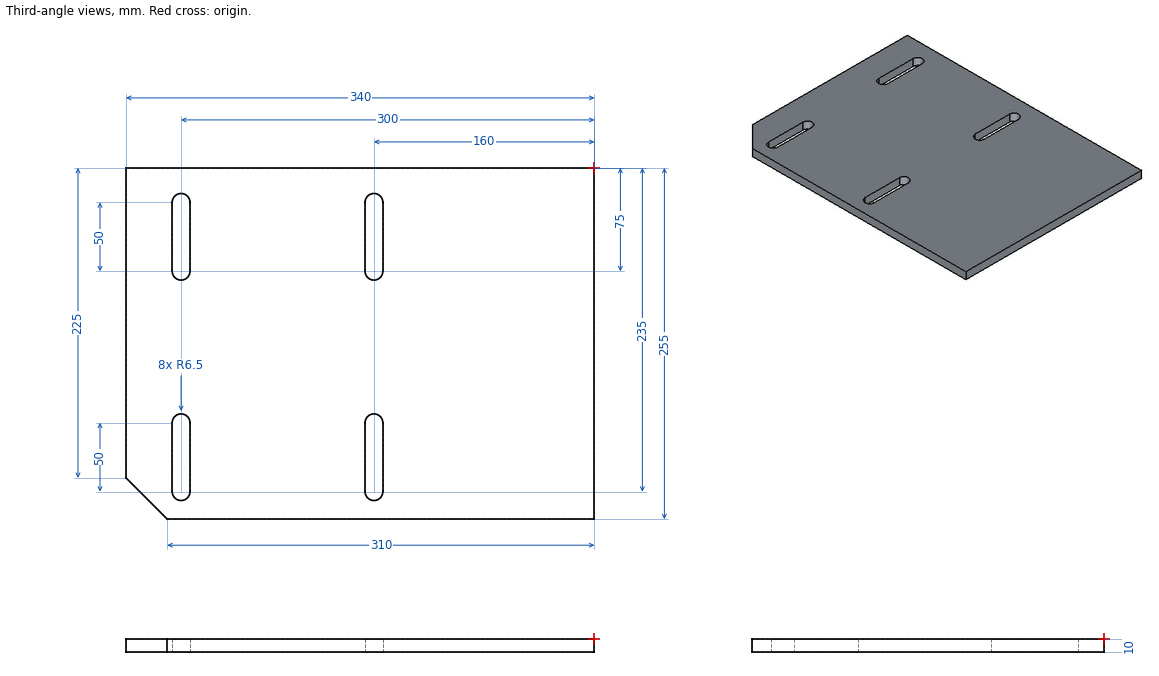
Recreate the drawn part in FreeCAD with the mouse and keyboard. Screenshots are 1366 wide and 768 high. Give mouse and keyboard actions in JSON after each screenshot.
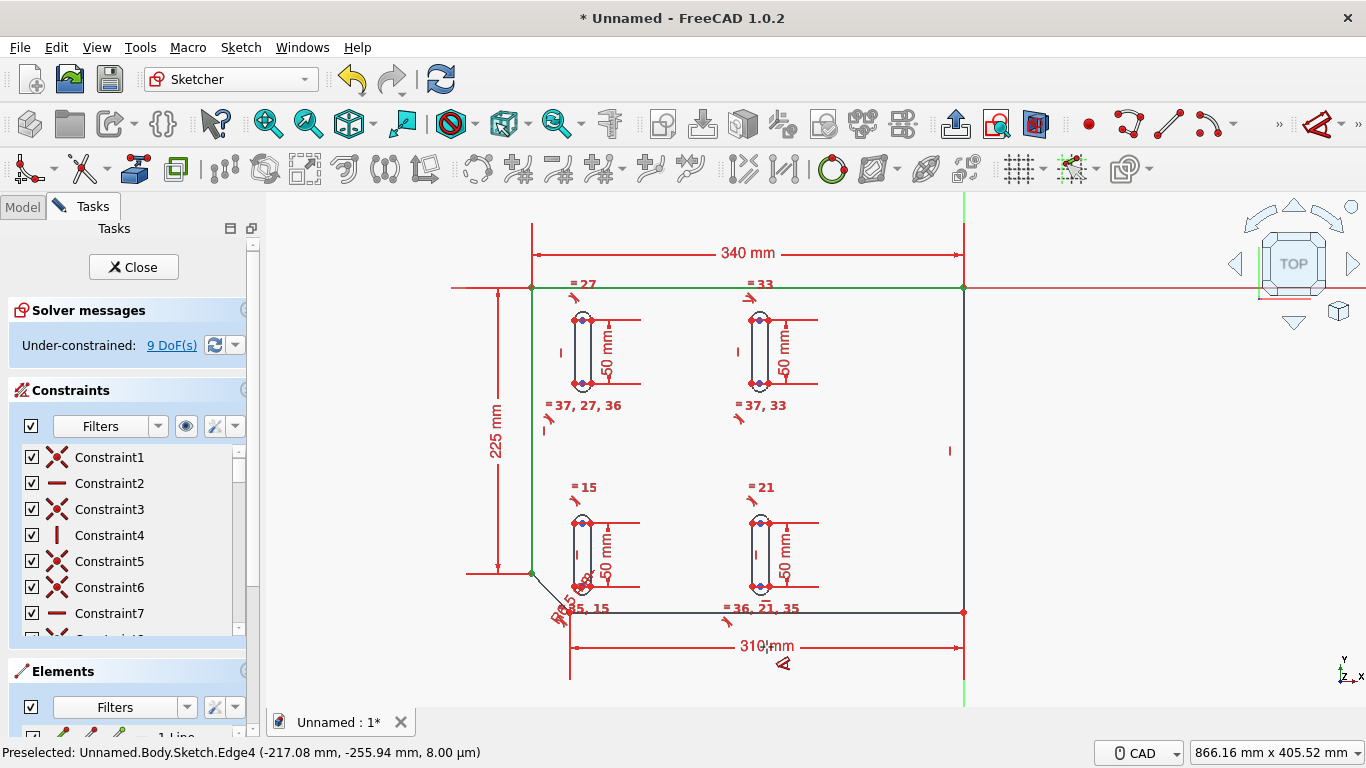
{"action": "left_click", "coordinate": [964, 515]}
{"action": "left_click", "coordinate": [998, 450]}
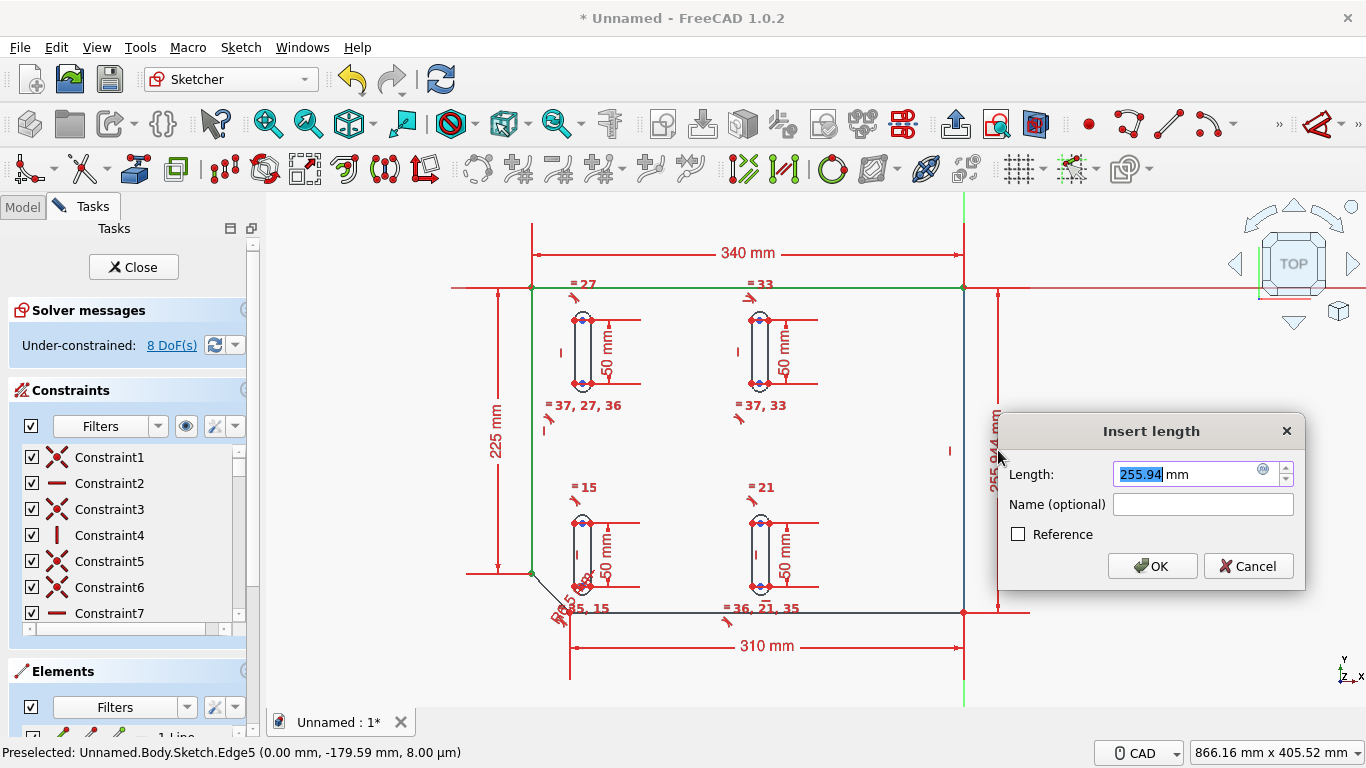
{"action": "type", "text": "255"}
{"action": "key", "text": "Return"}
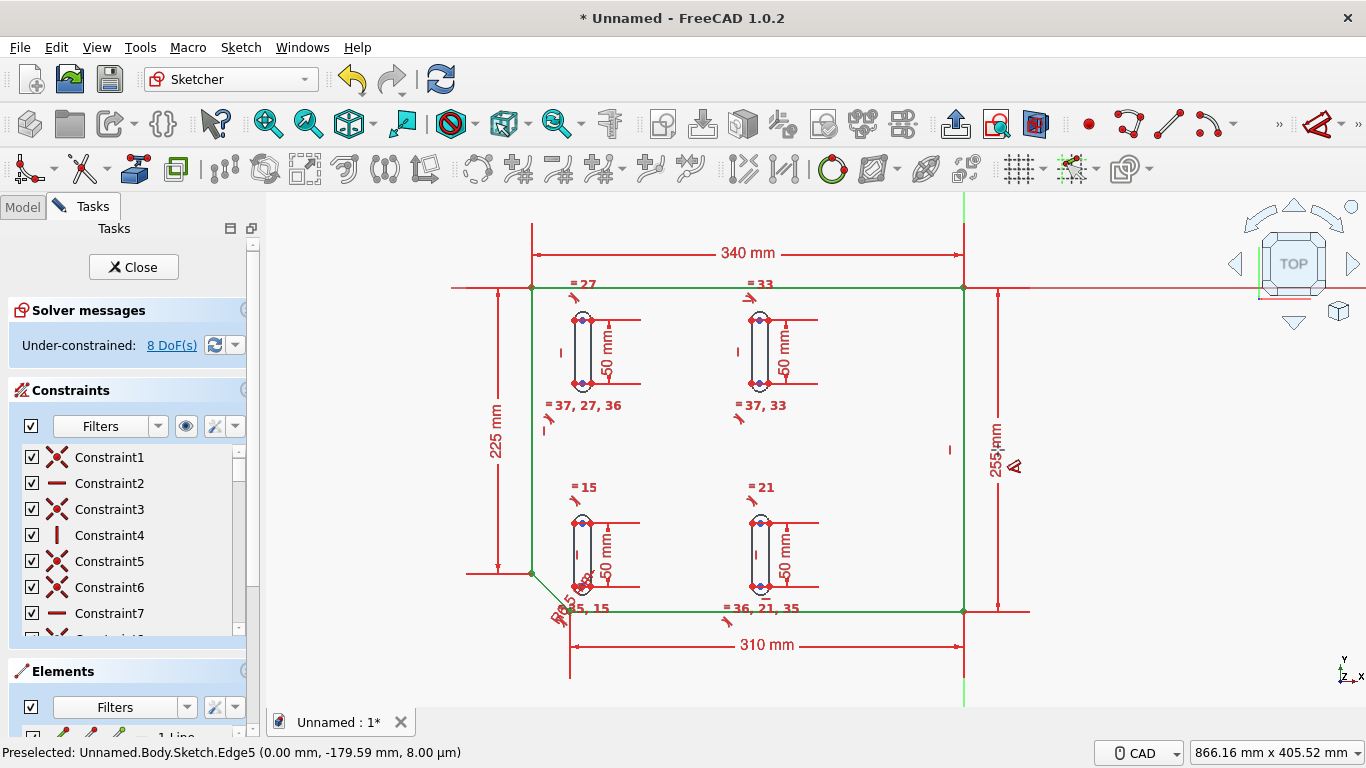
{"action": "scroll", "coordinate": [575, 384], "scroll_direction": "up", "scroll_amount": 2}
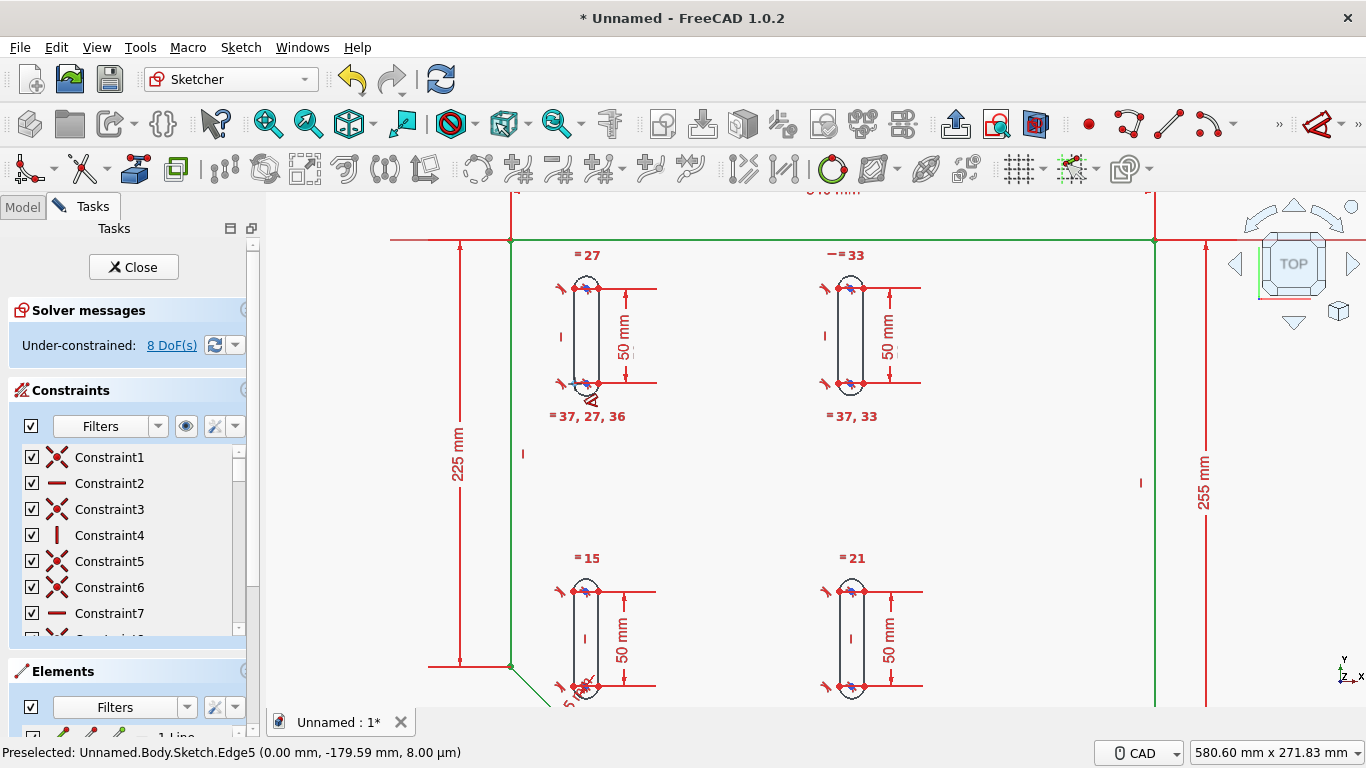
{"action": "left_click", "coordinate": [574, 383]}
{"action": "left_click", "coordinate": [1189, 312]}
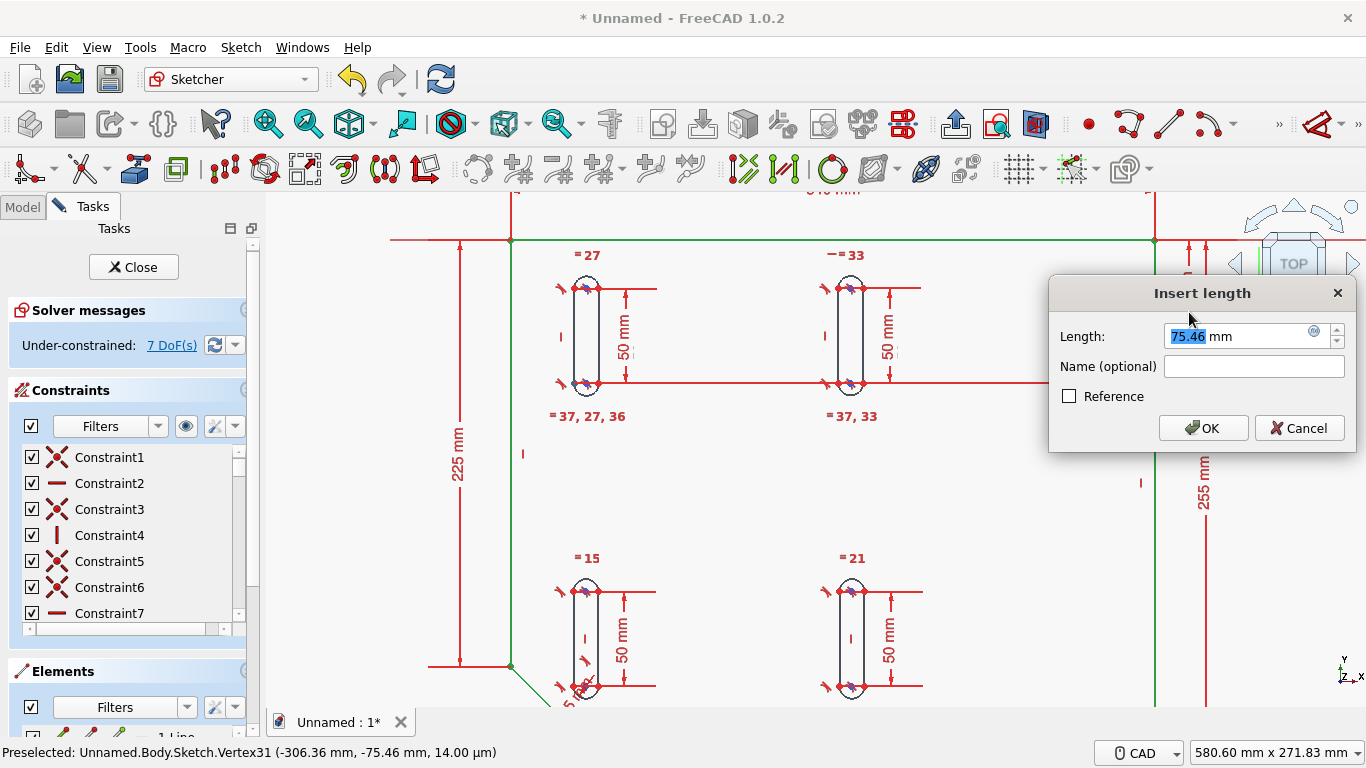
{"action": "type", "text": "75"}
{"action": "key", "text": "Return"}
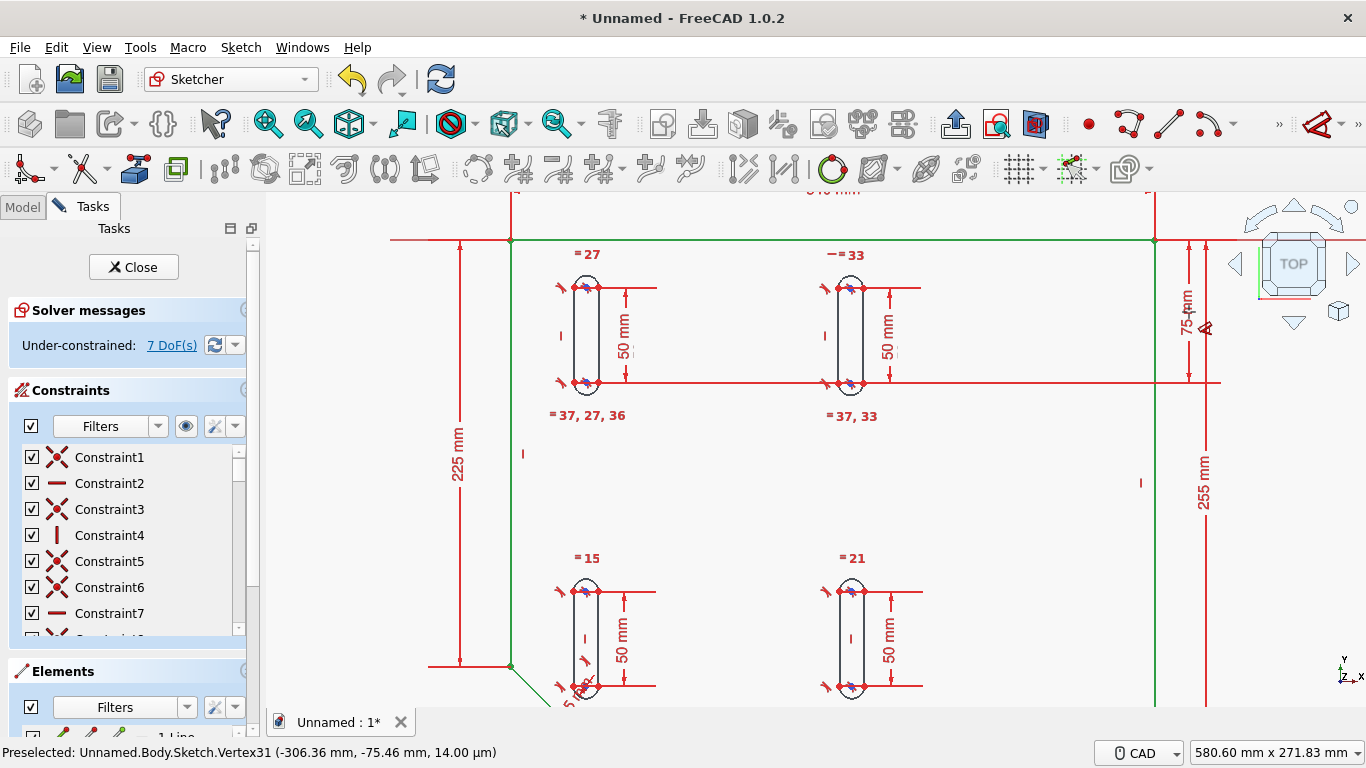
{"action": "left_click", "coordinate": [838, 383]}
{"action": "left_click", "coordinate": [1189, 279]}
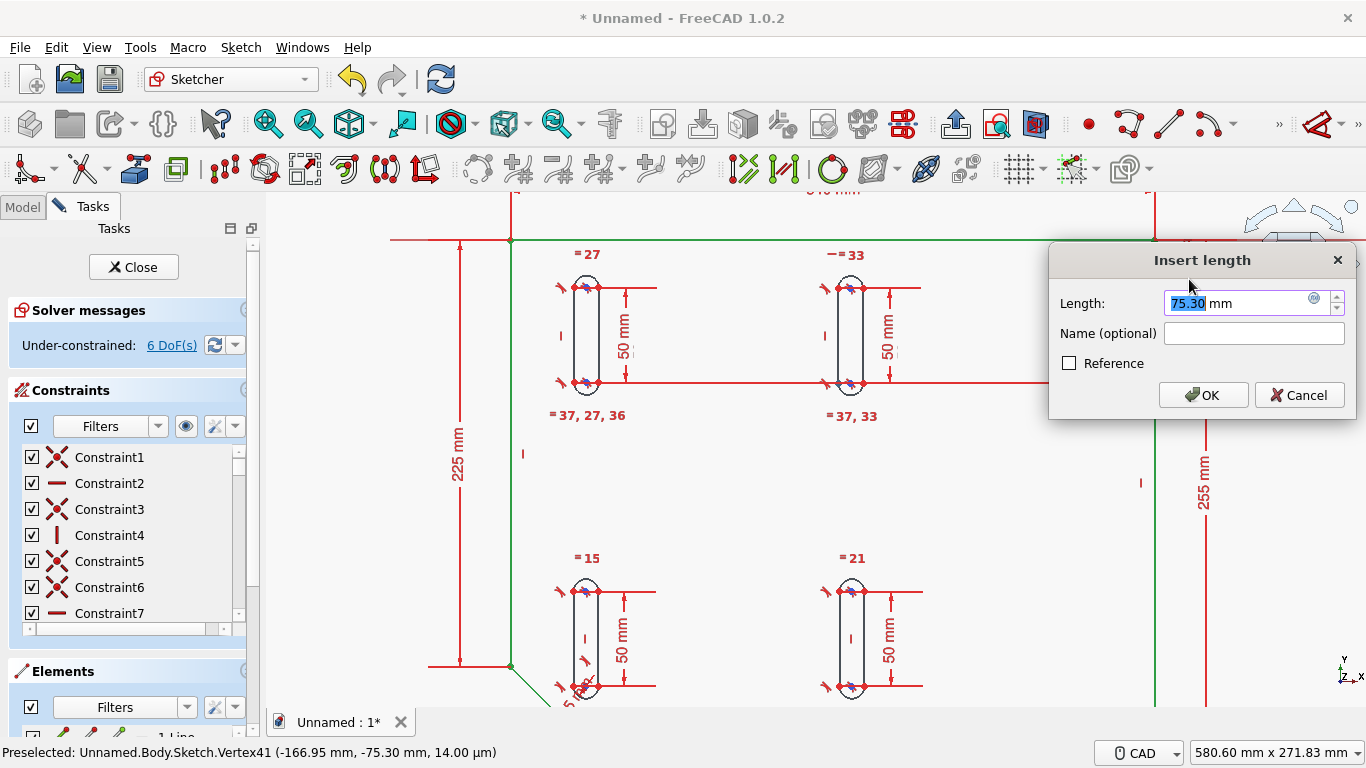
{"action": "type", "text": "75"}
{"action": "key", "text": "Return"}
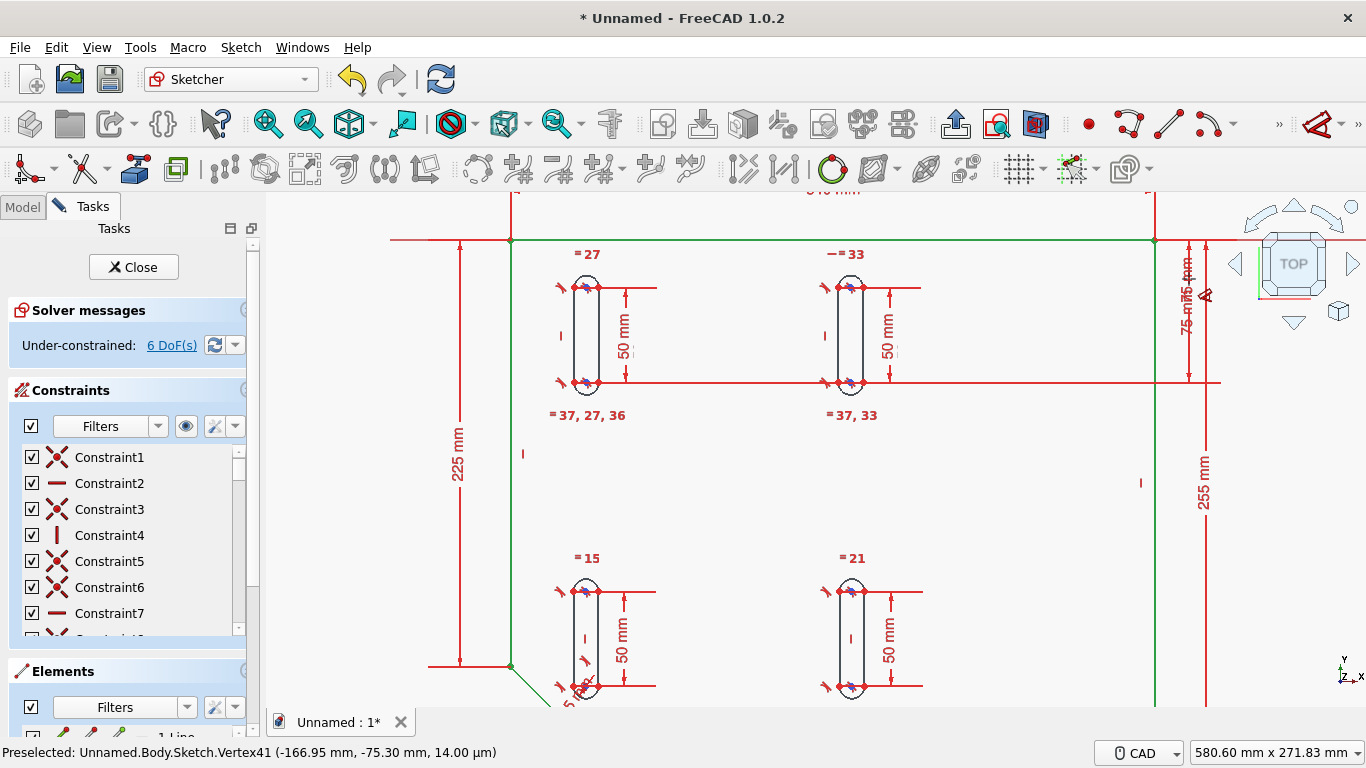
{"action": "scroll", "coordinate": [574, 383], "scroll_direction": "down", "scroll_amount": 2}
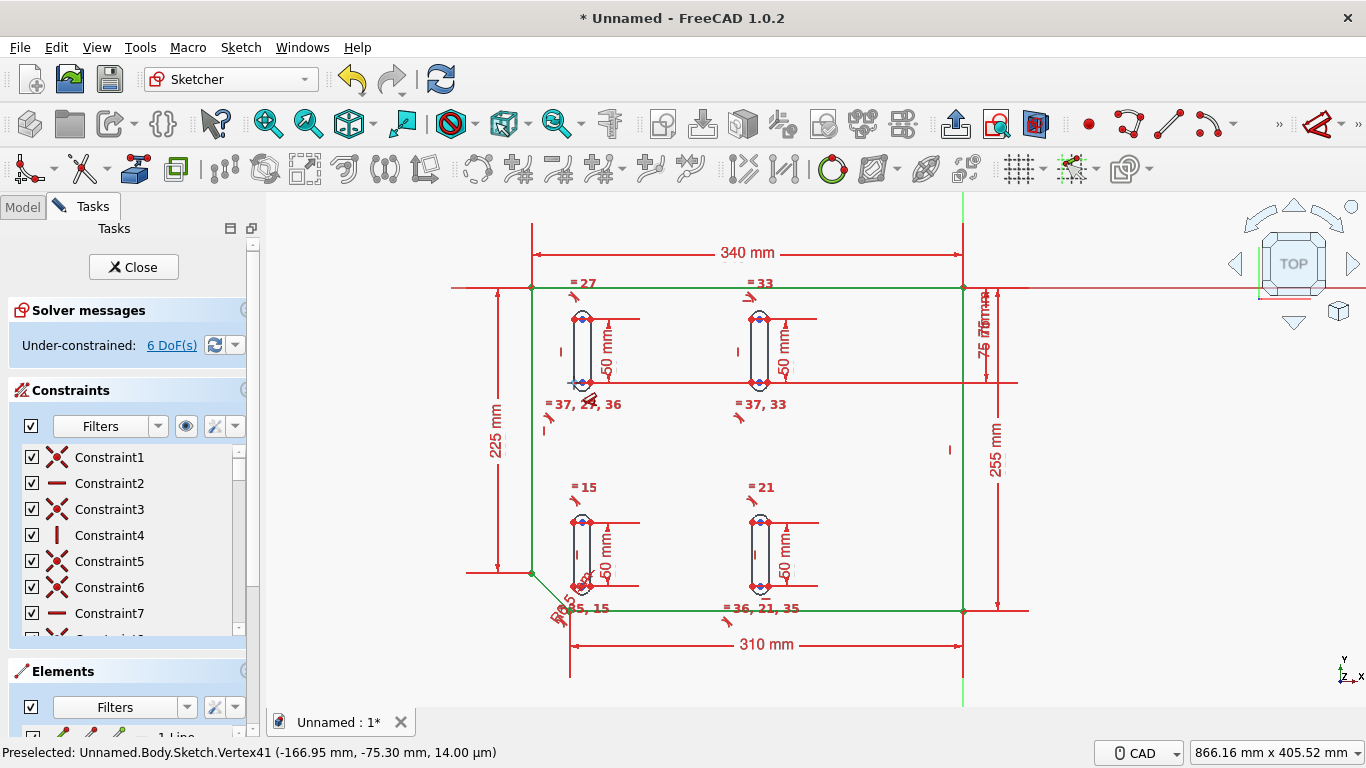
{"action": "scroll", "coordinate": [574, 586], "scroll_direction": "up", "scroll_amount": 2}